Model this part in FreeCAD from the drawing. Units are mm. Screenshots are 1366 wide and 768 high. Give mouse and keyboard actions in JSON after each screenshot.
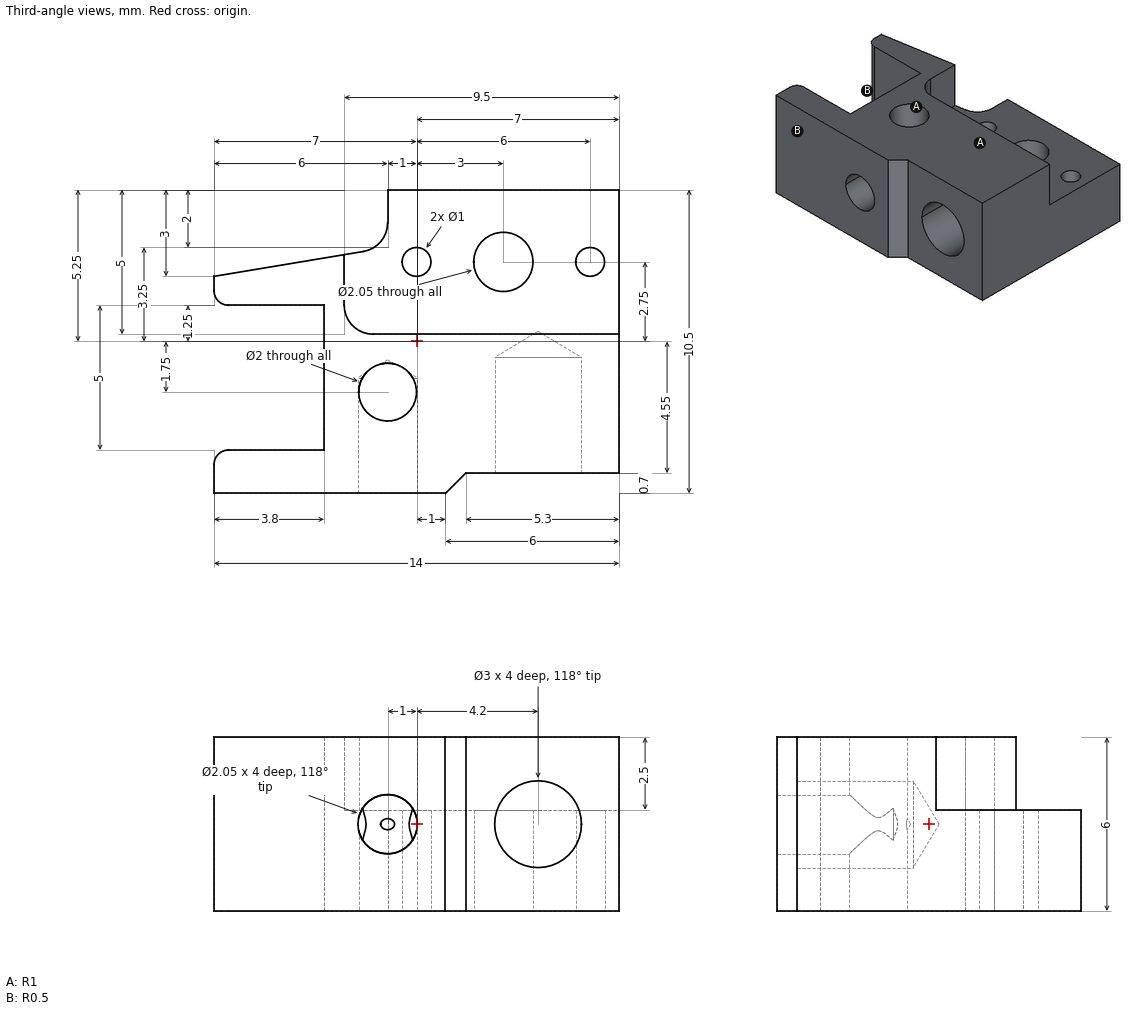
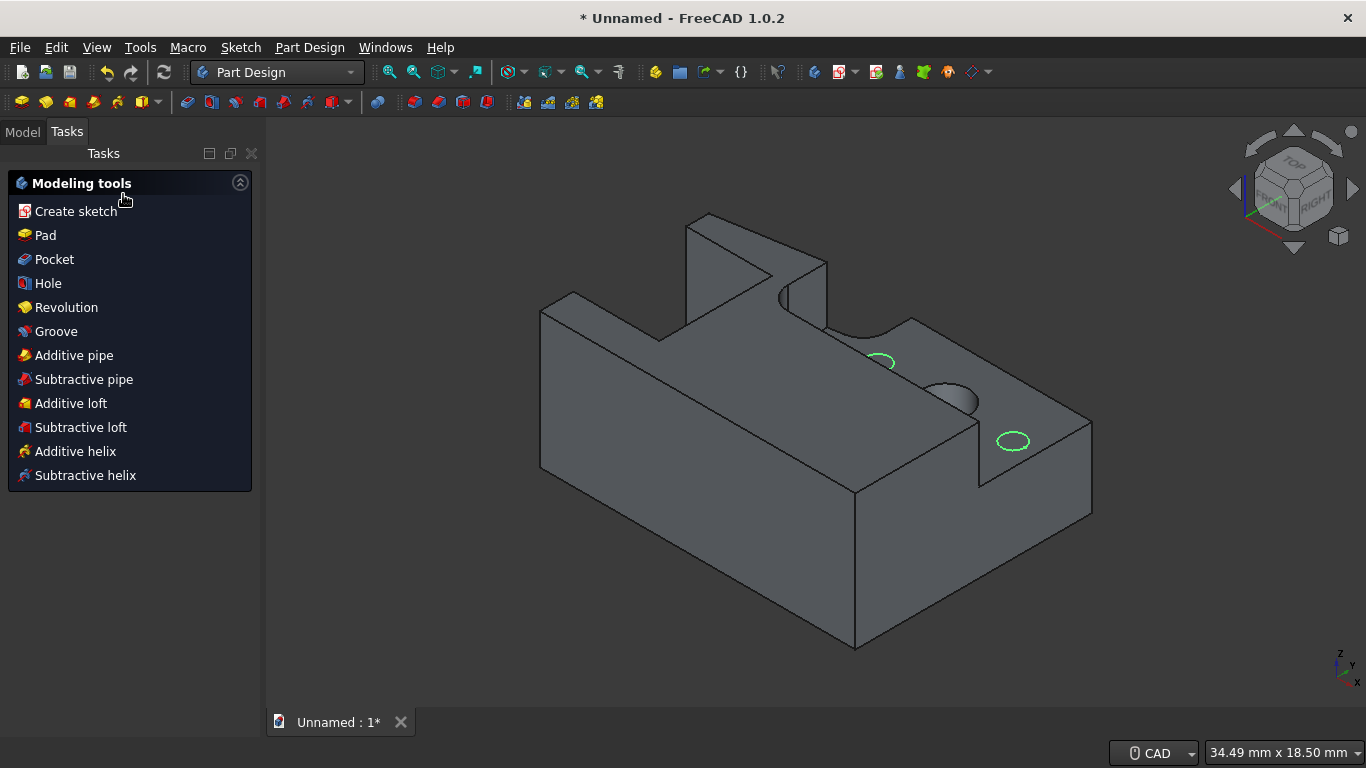
{"action": "left_click", "coordinate": [188, 102]}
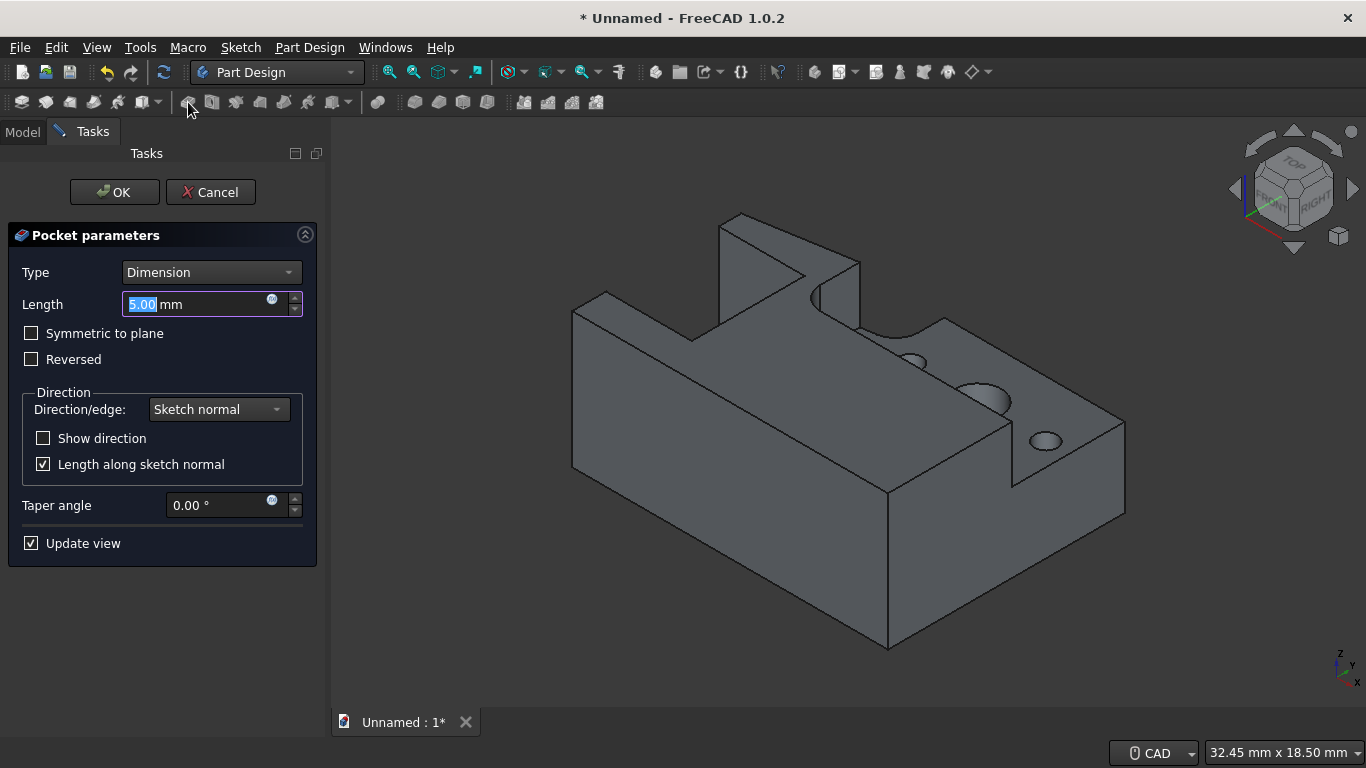
{"action": "left_click", "coordinate": [212, 272]}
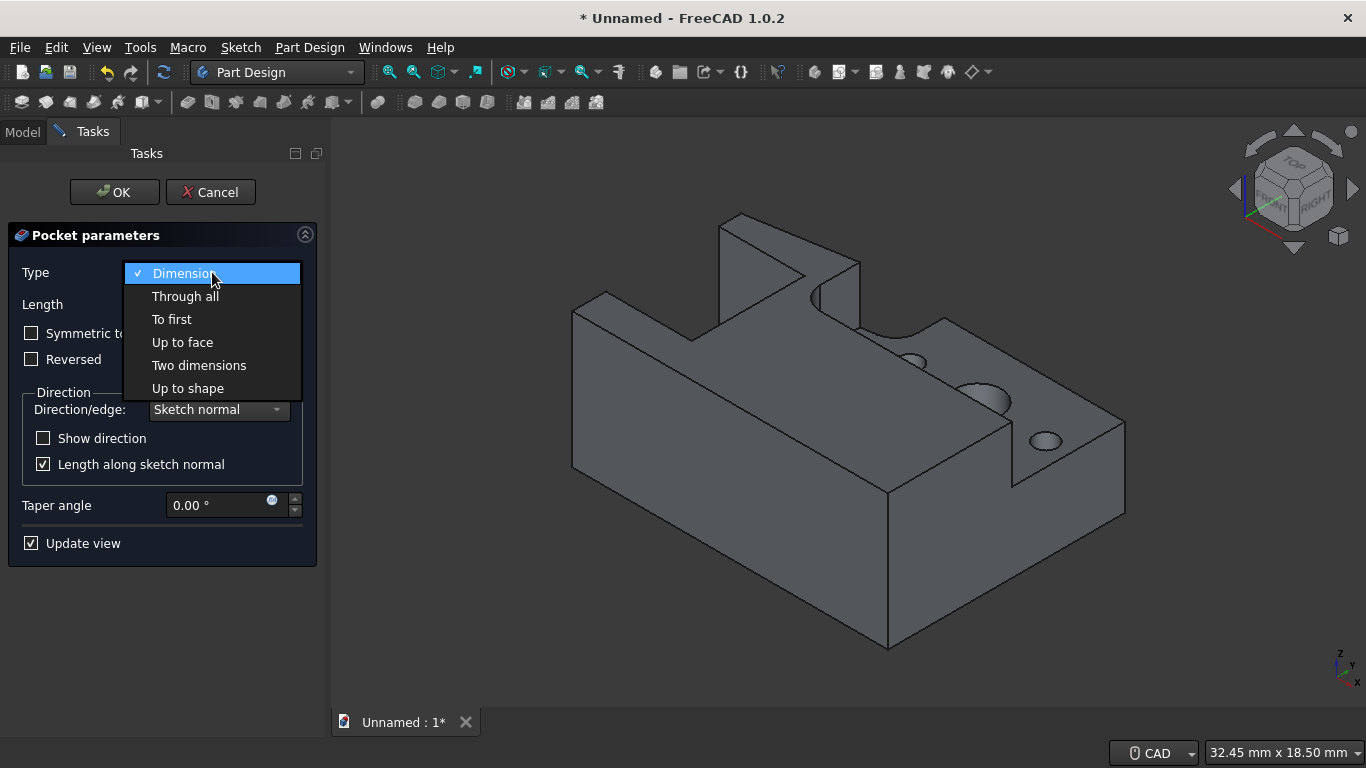
{"action": "left_click", "coordinate": [212, 296]}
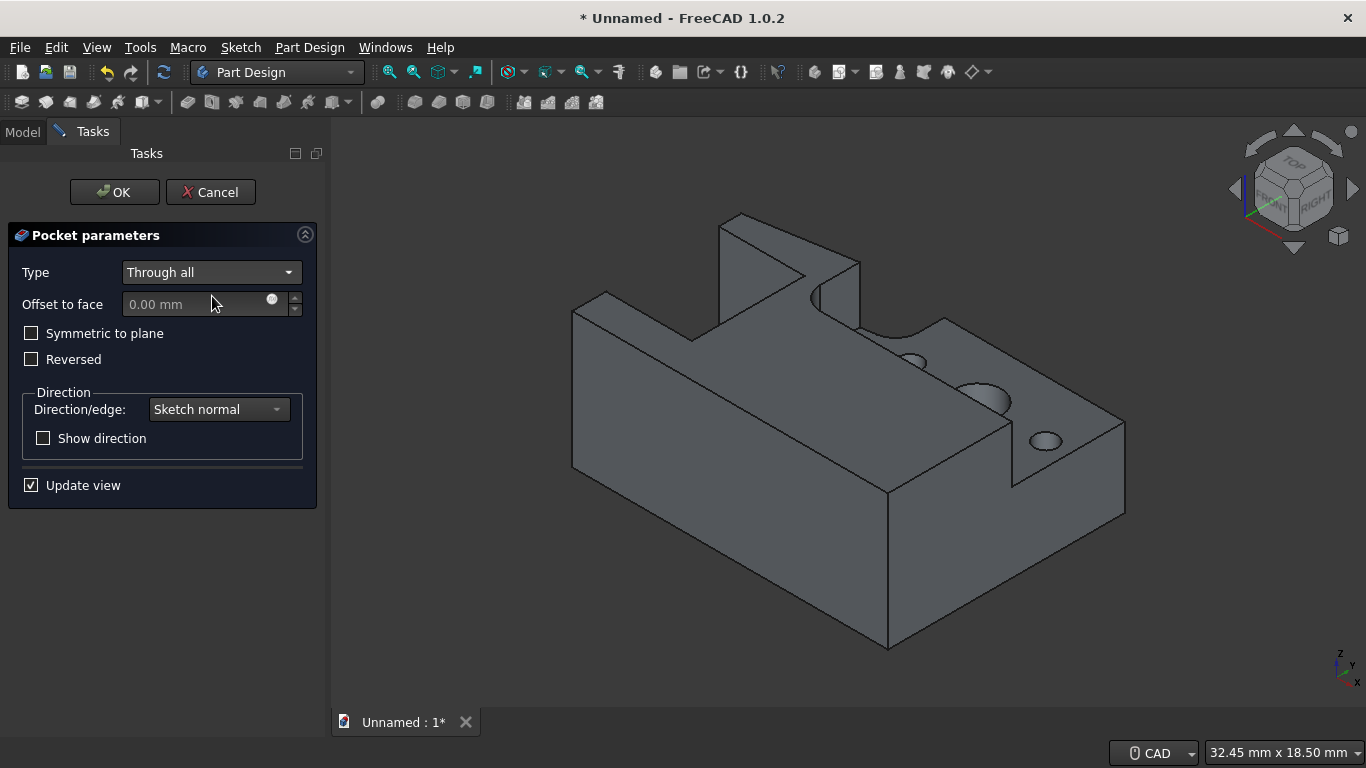
{"action": "left_click", "coordinate": [115, 192]}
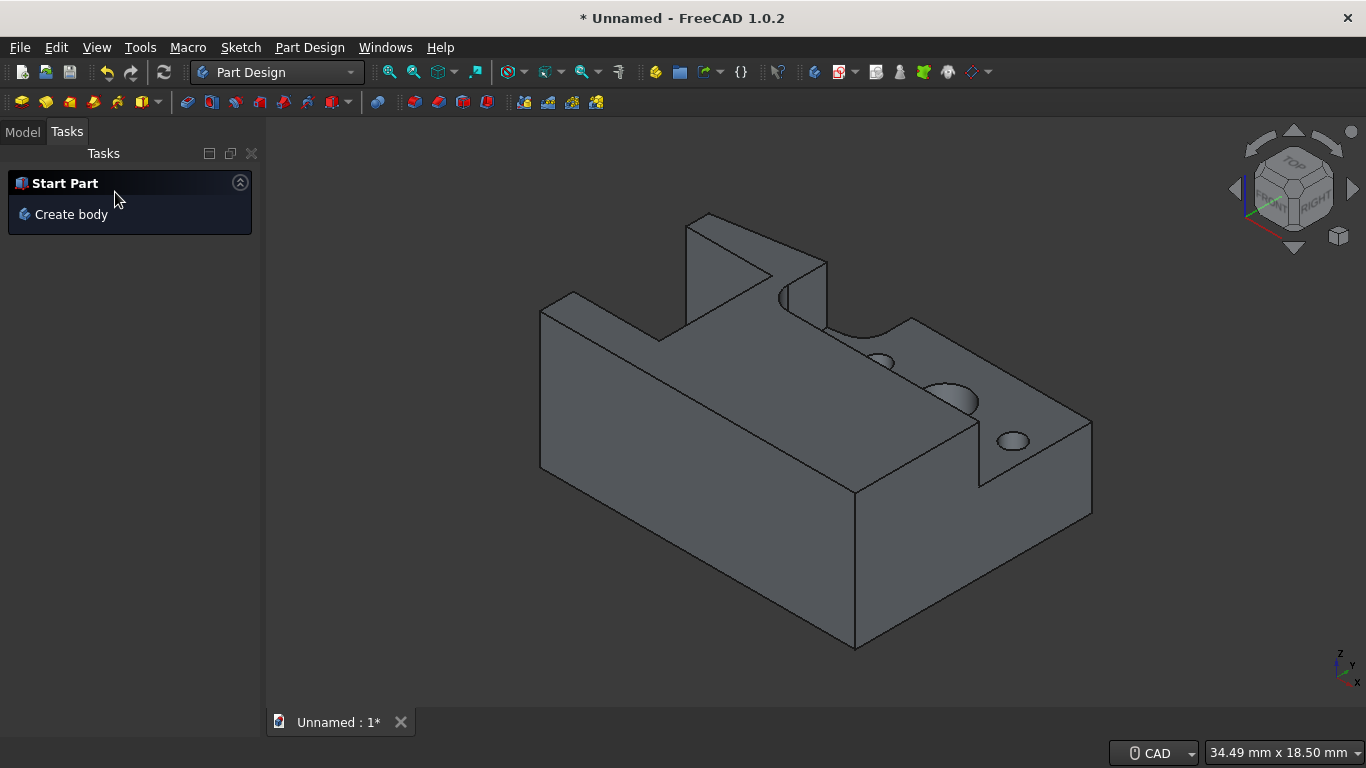
{"action": "left_click", "coordinate": [854, 415]}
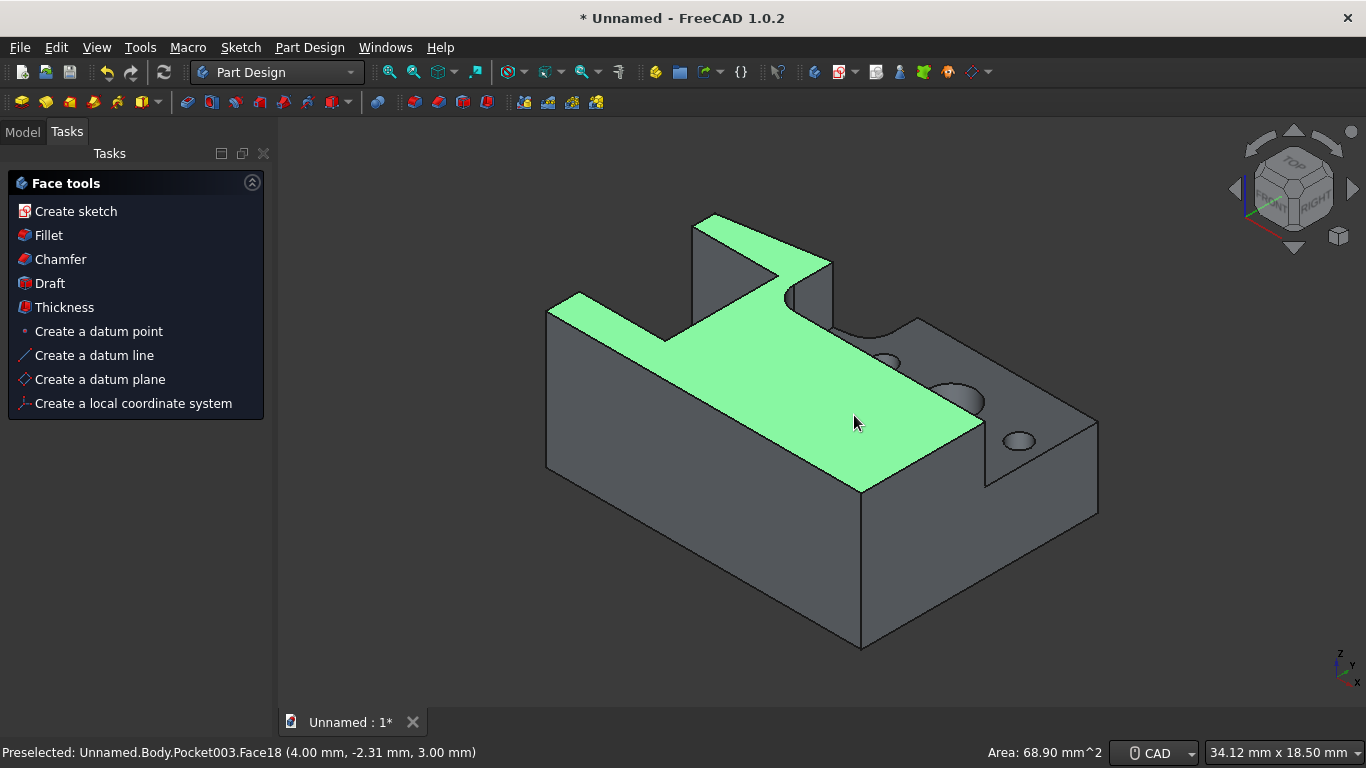
{"action": "left_click", "coordinate": [840, 72]}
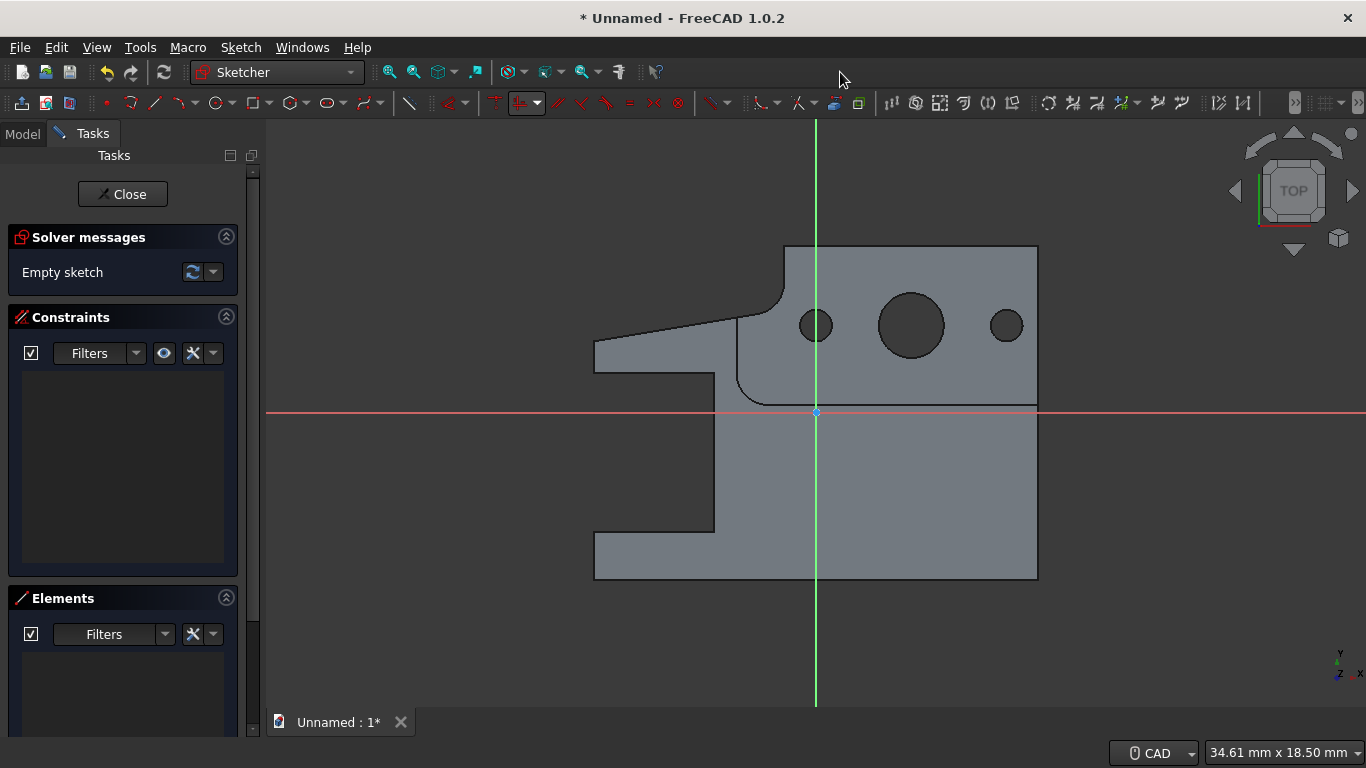
{"action": "scroll", "coordinate": [796, 471], "scroll_direction": "up", "scroll_amount": 7}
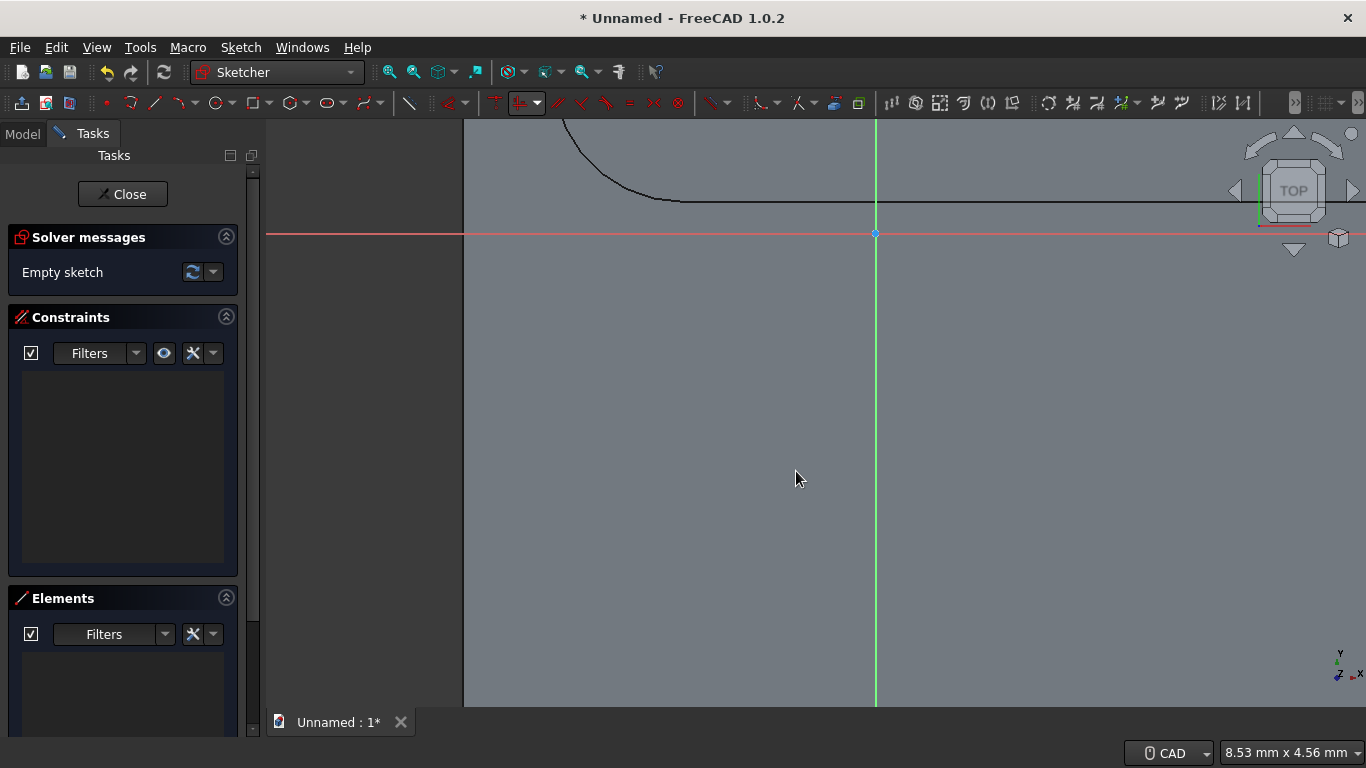
{"action": "left_click", "coordinate": [216, 104]}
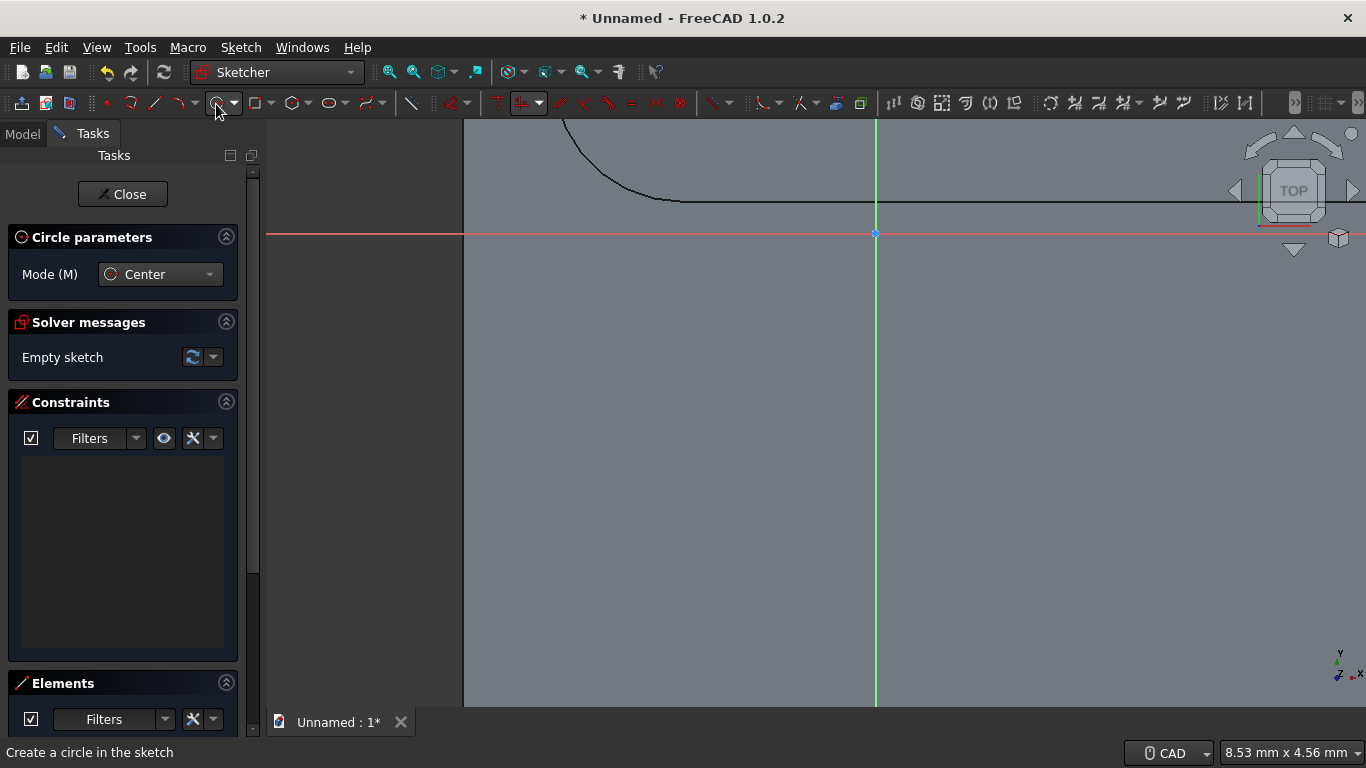
{"action": "left_click", "coordinate": [747, 460]}
{"action": "left_click", "coordinate": [838, 368]}
{"action": "key", "text": "Escape"}